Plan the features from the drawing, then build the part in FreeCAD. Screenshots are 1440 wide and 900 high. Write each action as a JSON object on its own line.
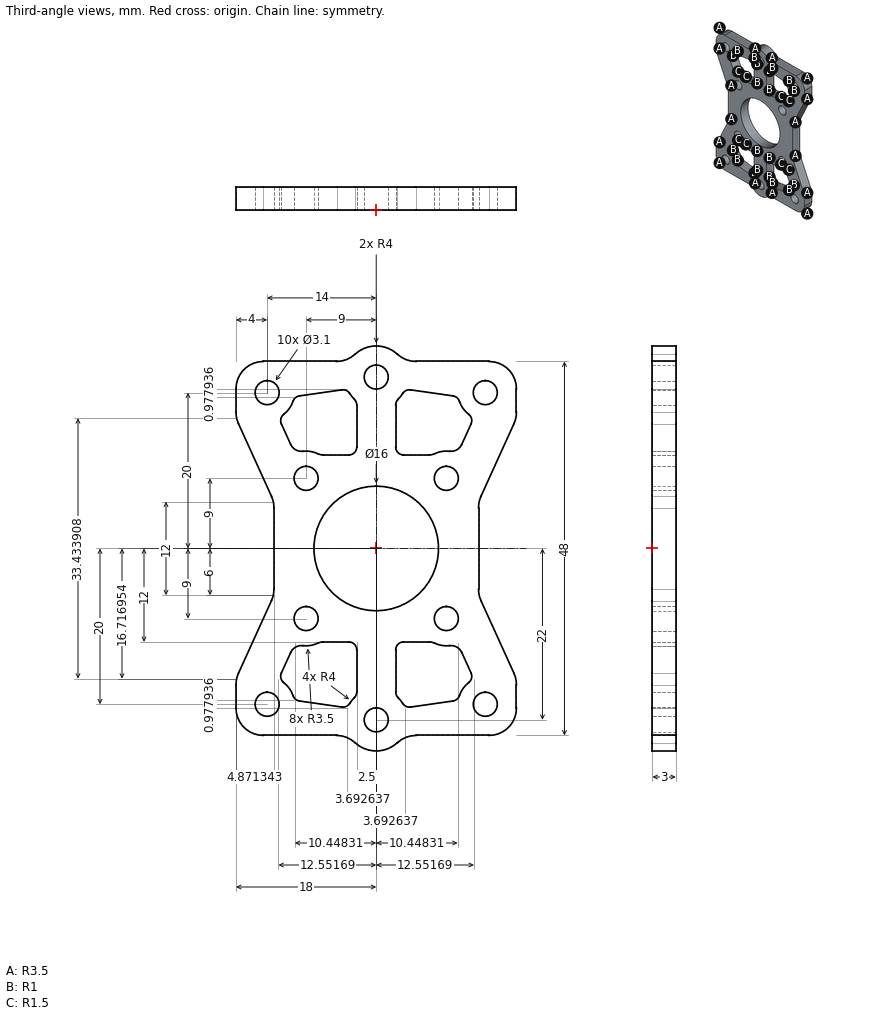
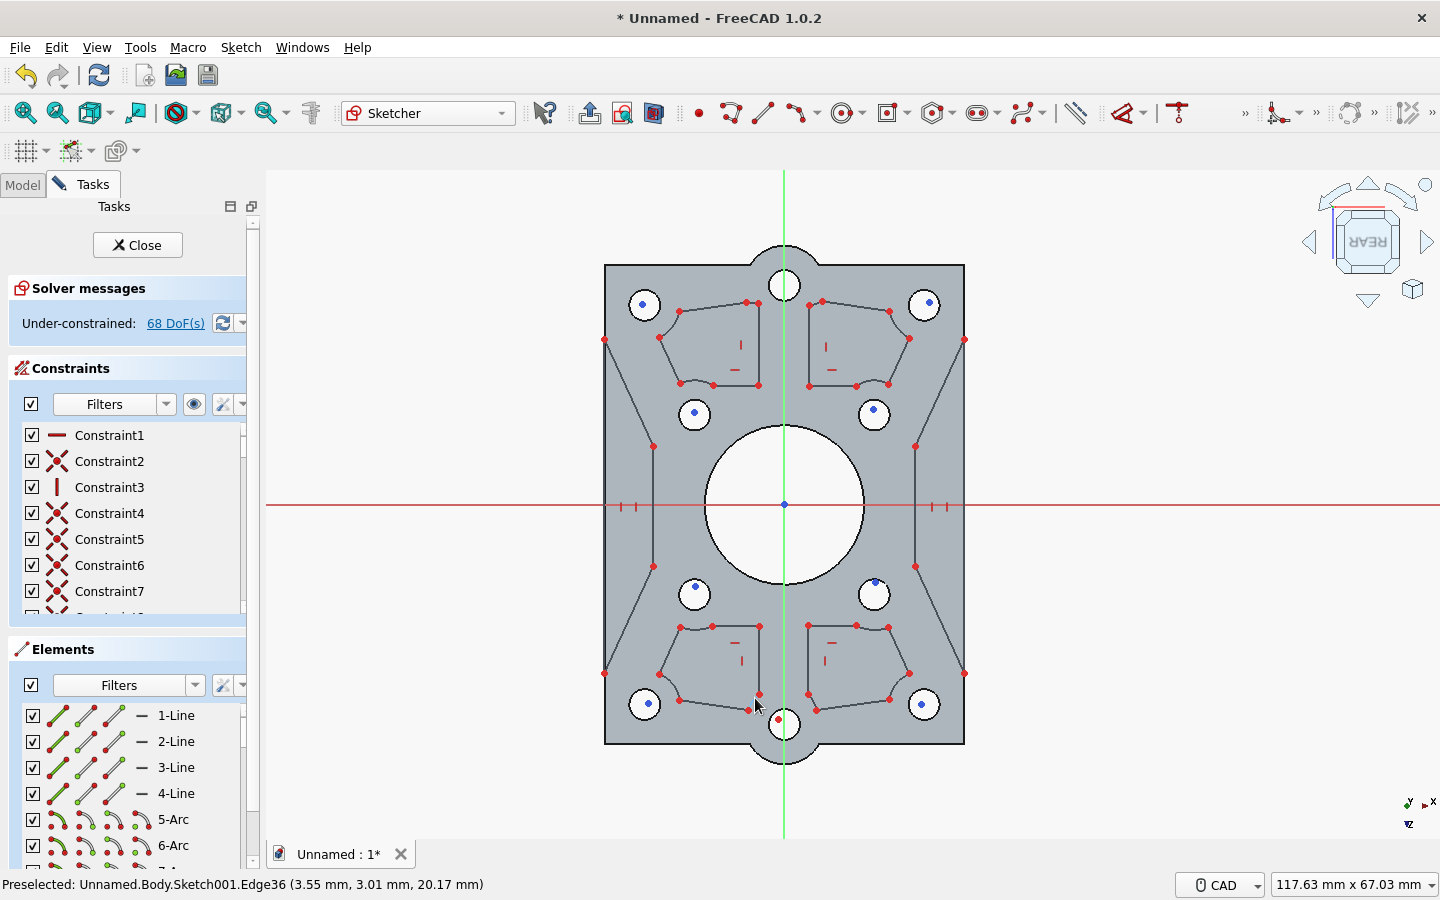
{"action": "scroll", "coordinate": [704, 382], "scroll_direction": "up", "scroll_amount": 2}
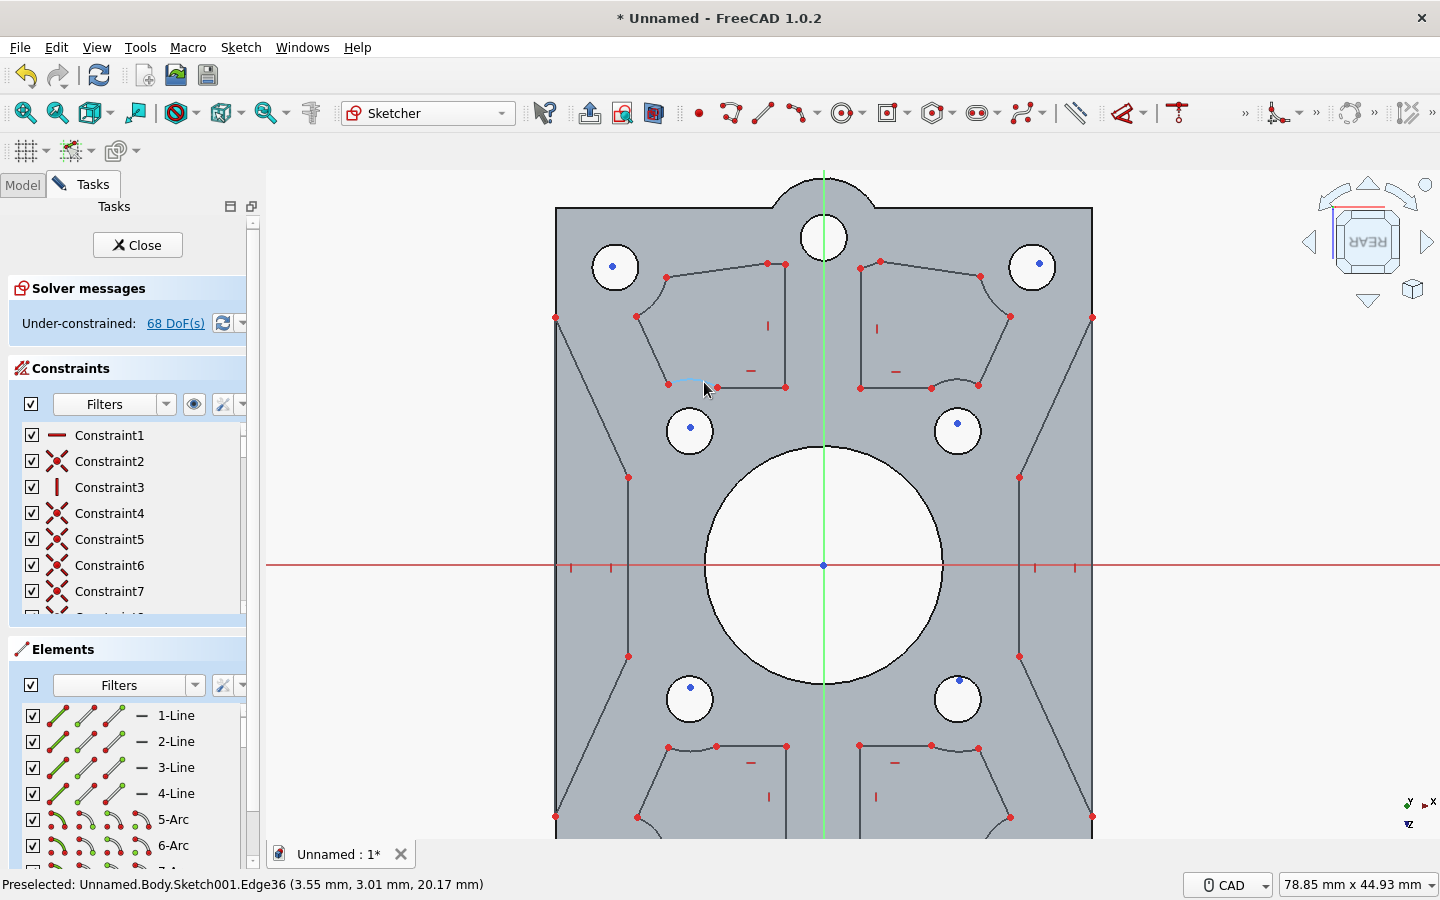
{"action": "left_click", "coordinate": [703, 381]}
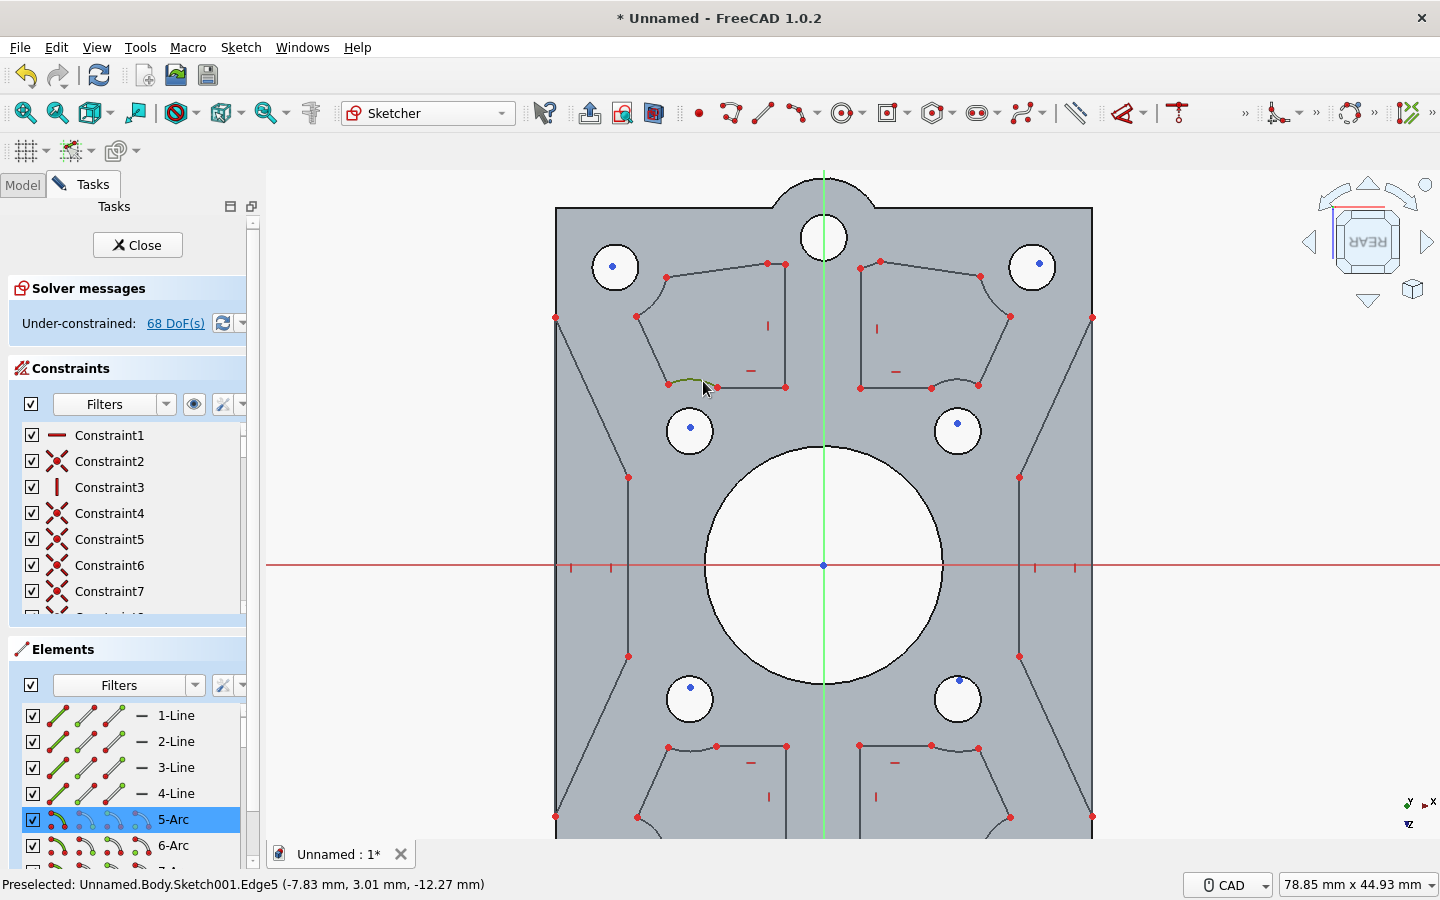
{"action": "left_click", "coordinate": [649, 308]}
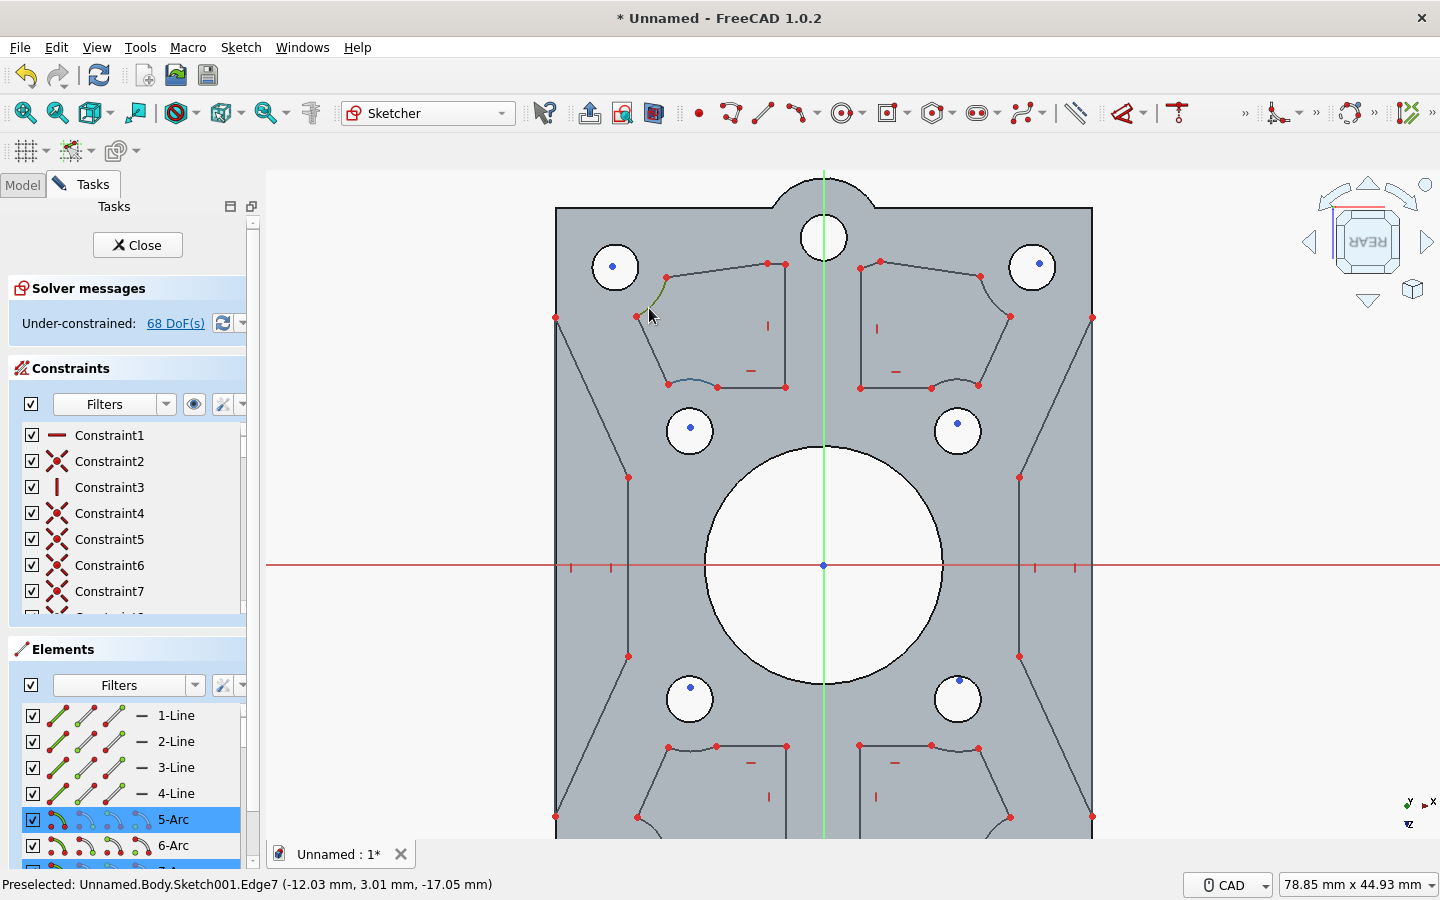
{"action": "left_click", "coordinate": [965, 380]}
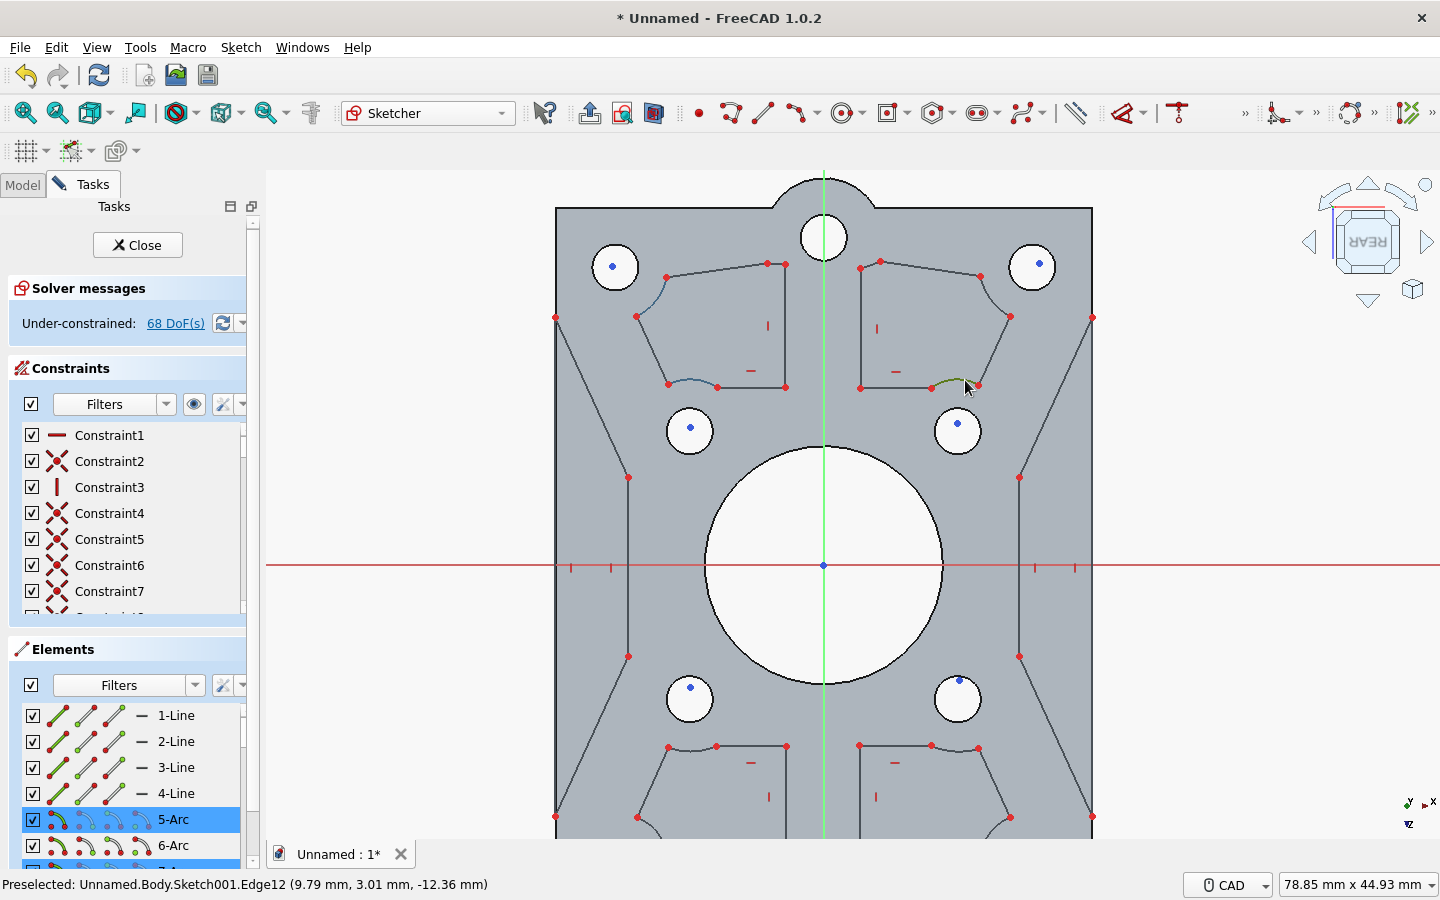
{"action": "left_click", "coordinate": [986, 291]}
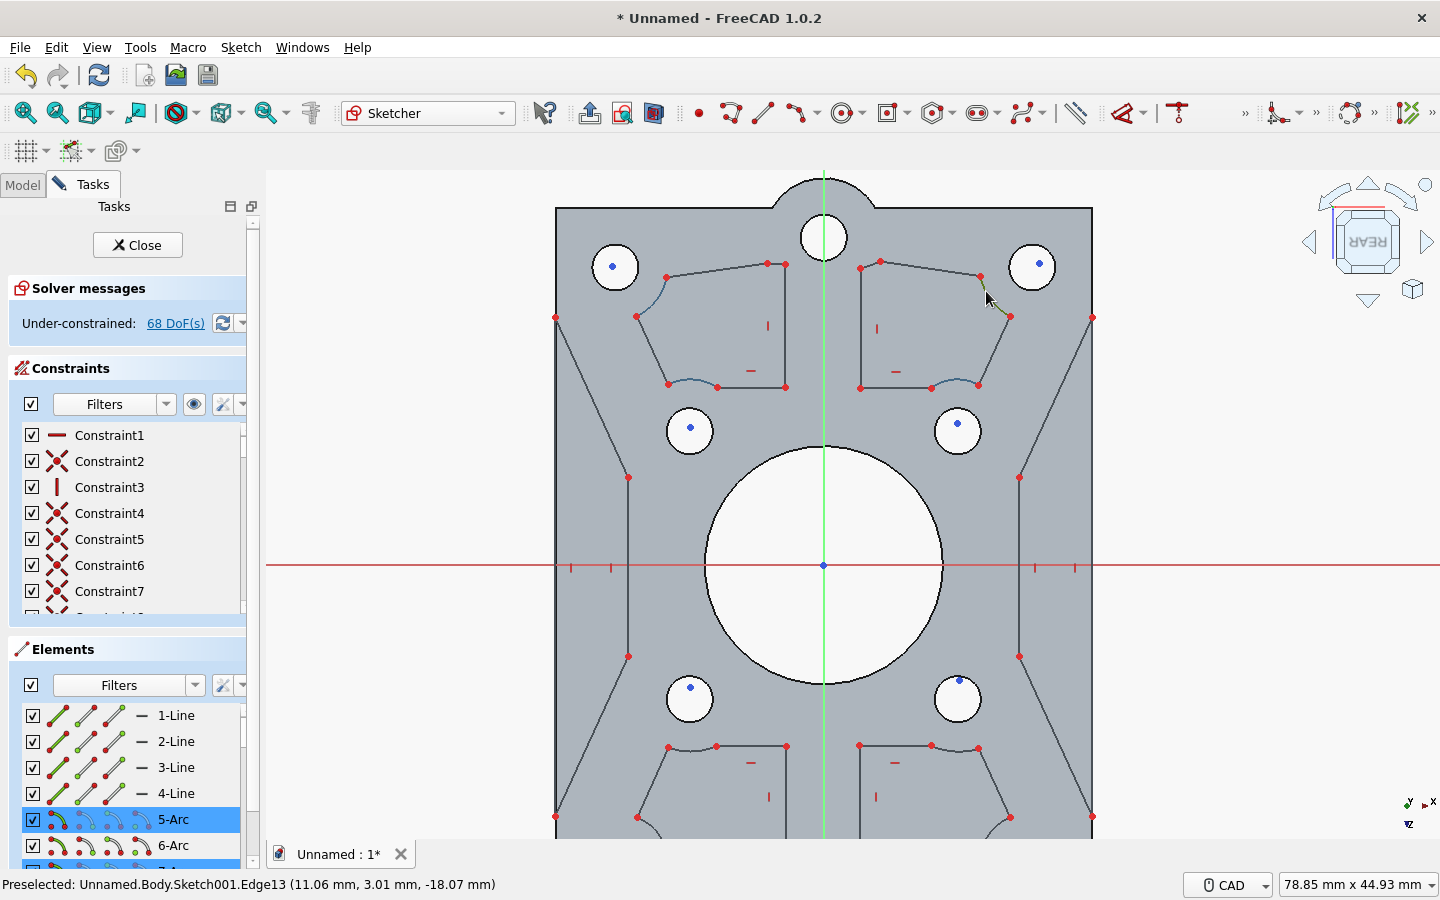
{"action": "left_click", "coordinate": [683, 751]}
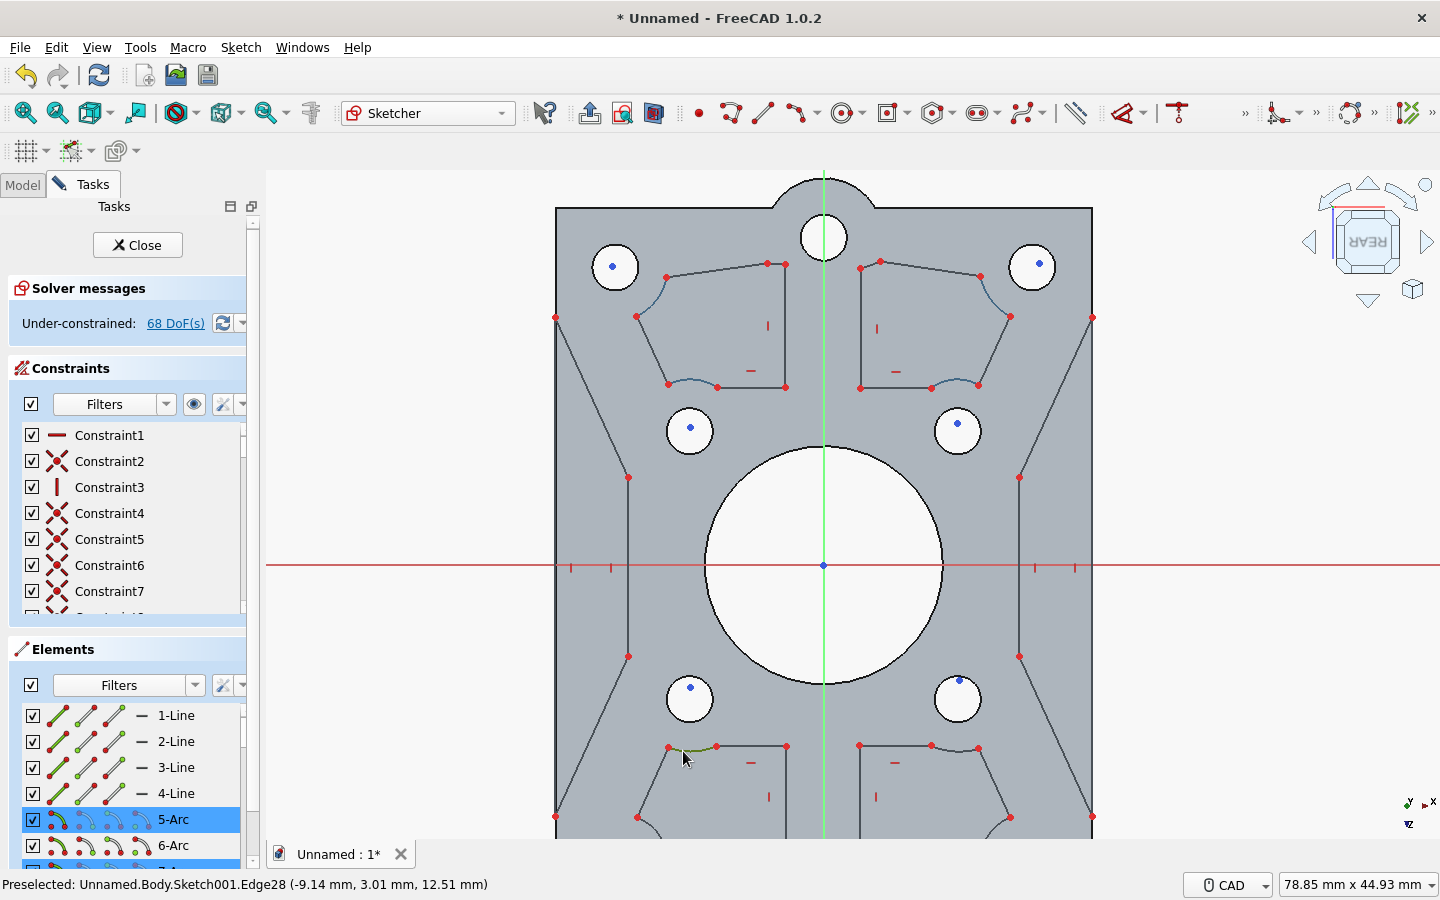
{"action": "scroll", "coordinate": [705, 381], "scroll_direction": "down", "scroll_amount": 2}